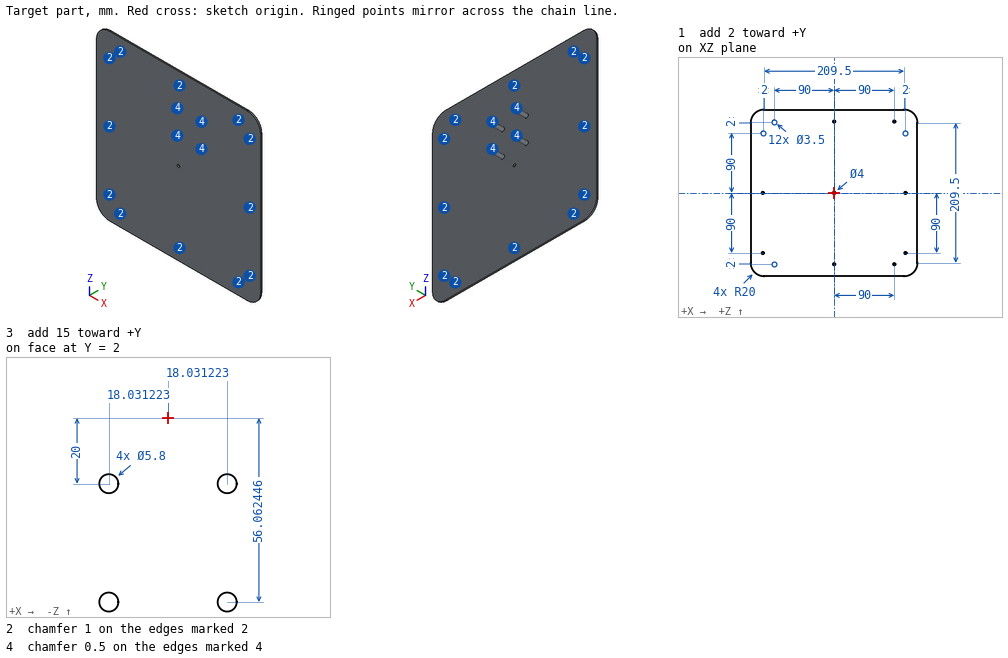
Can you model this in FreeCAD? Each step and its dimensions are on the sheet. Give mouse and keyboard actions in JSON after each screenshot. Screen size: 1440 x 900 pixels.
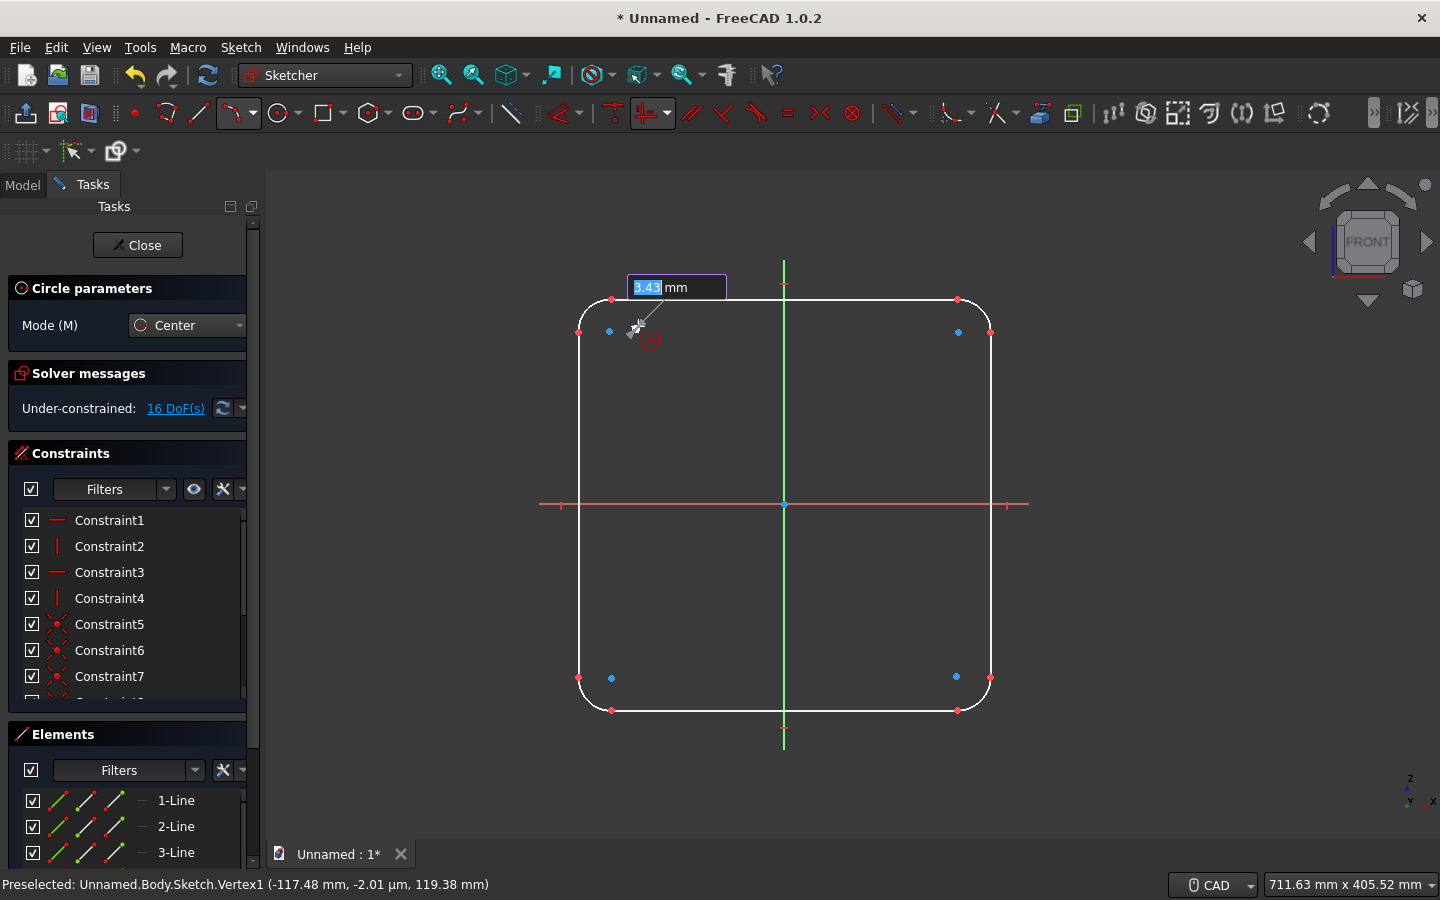
{"action": "type", "text": "3.5"}
{"action": "key", "text": "Return"}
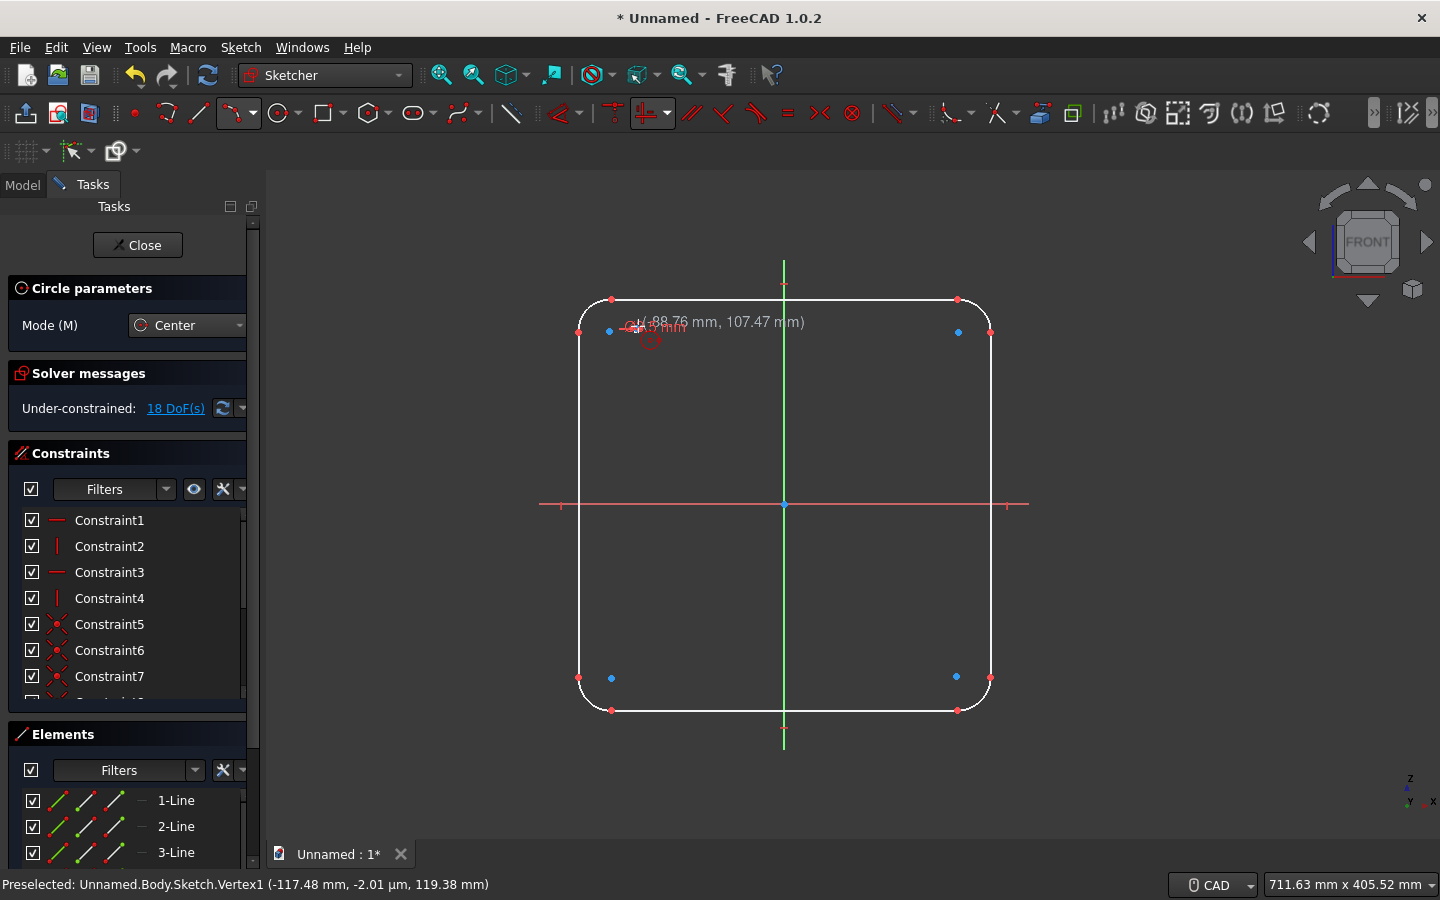
{"action": "scroll", "coordinate": [608, 356], "scroll_direction": "up", "scroll_amount": 11}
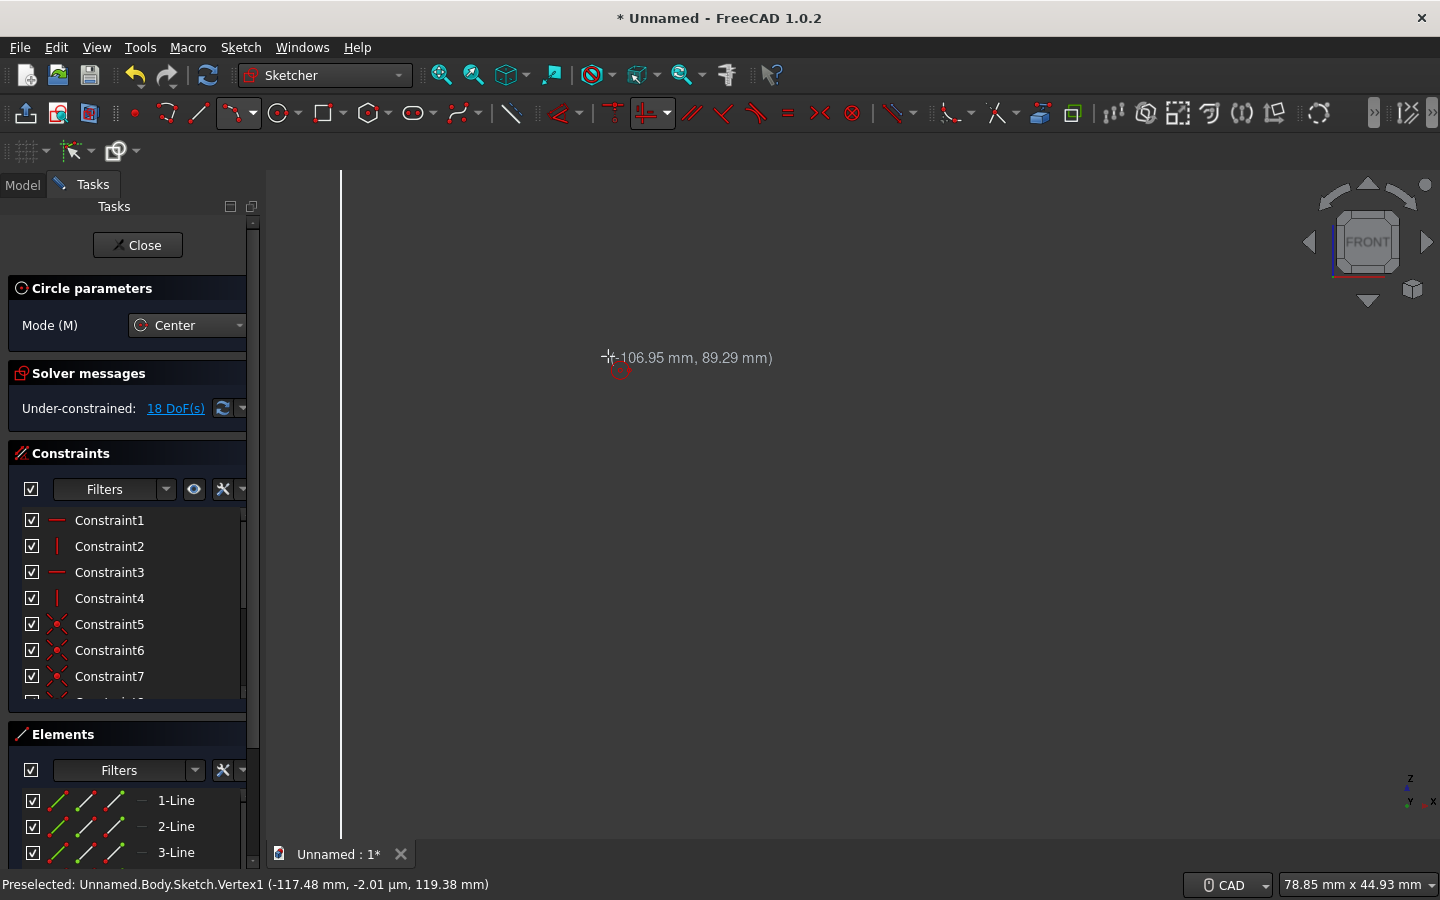
{"action": "scroll", "coordinate": [608, 357], "scroll_direction": "down", "scroll_amount": 11}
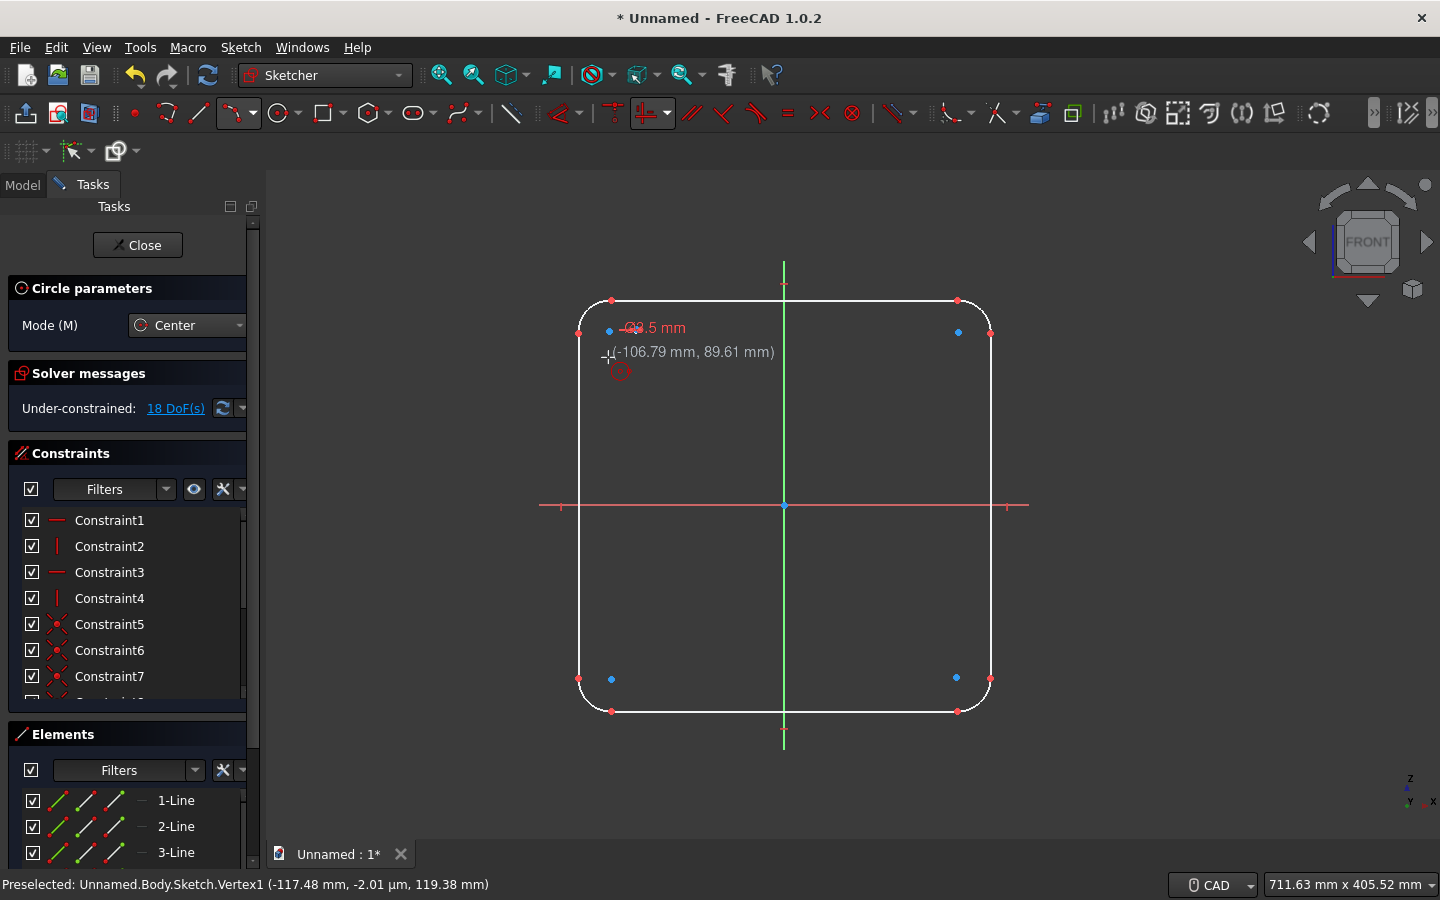
{"action": "left_click", "coordinate": [608, 357]}
{"action": "mouse_move", "coordinate": [610, 355]}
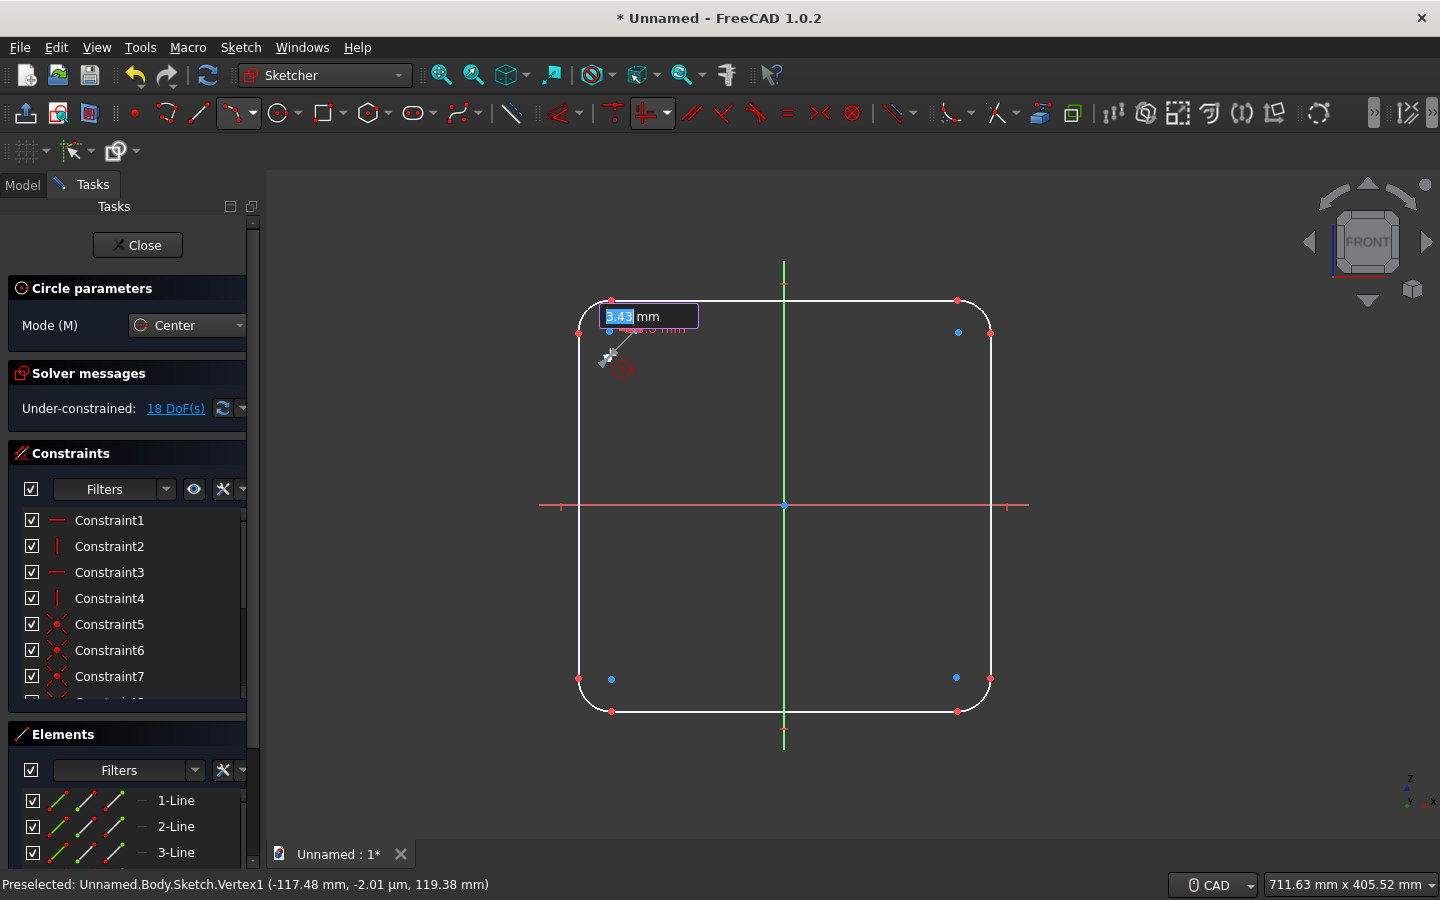
{"action": "type", "text": "3.5"}
{"action": "key", "text": "Return"}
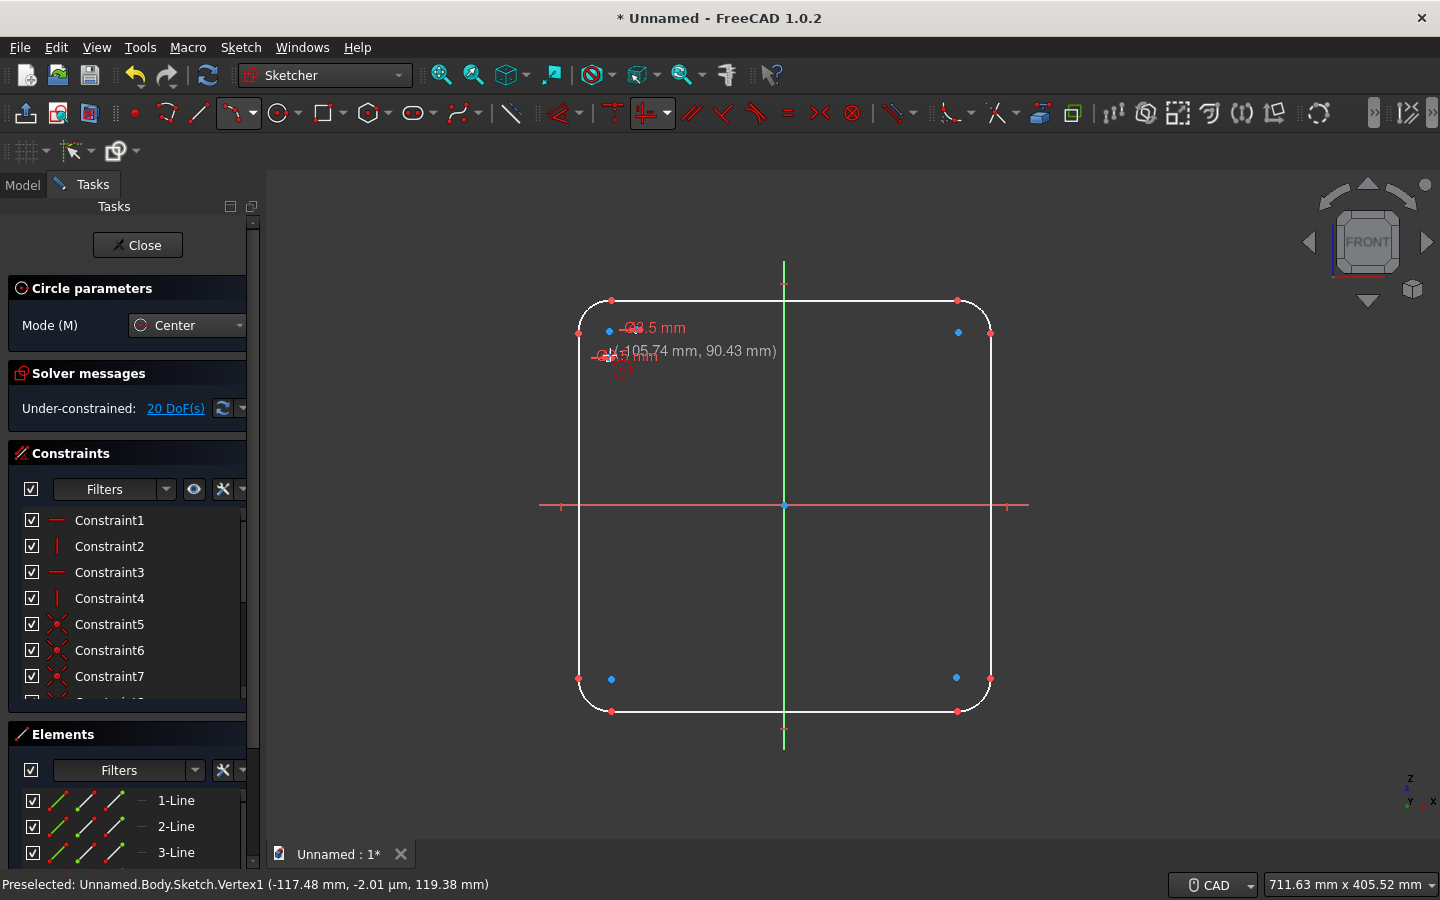
{"action": "scroll", "coordinate": [784, 329], "scroll_direction": "up", "scroll_amount": 11}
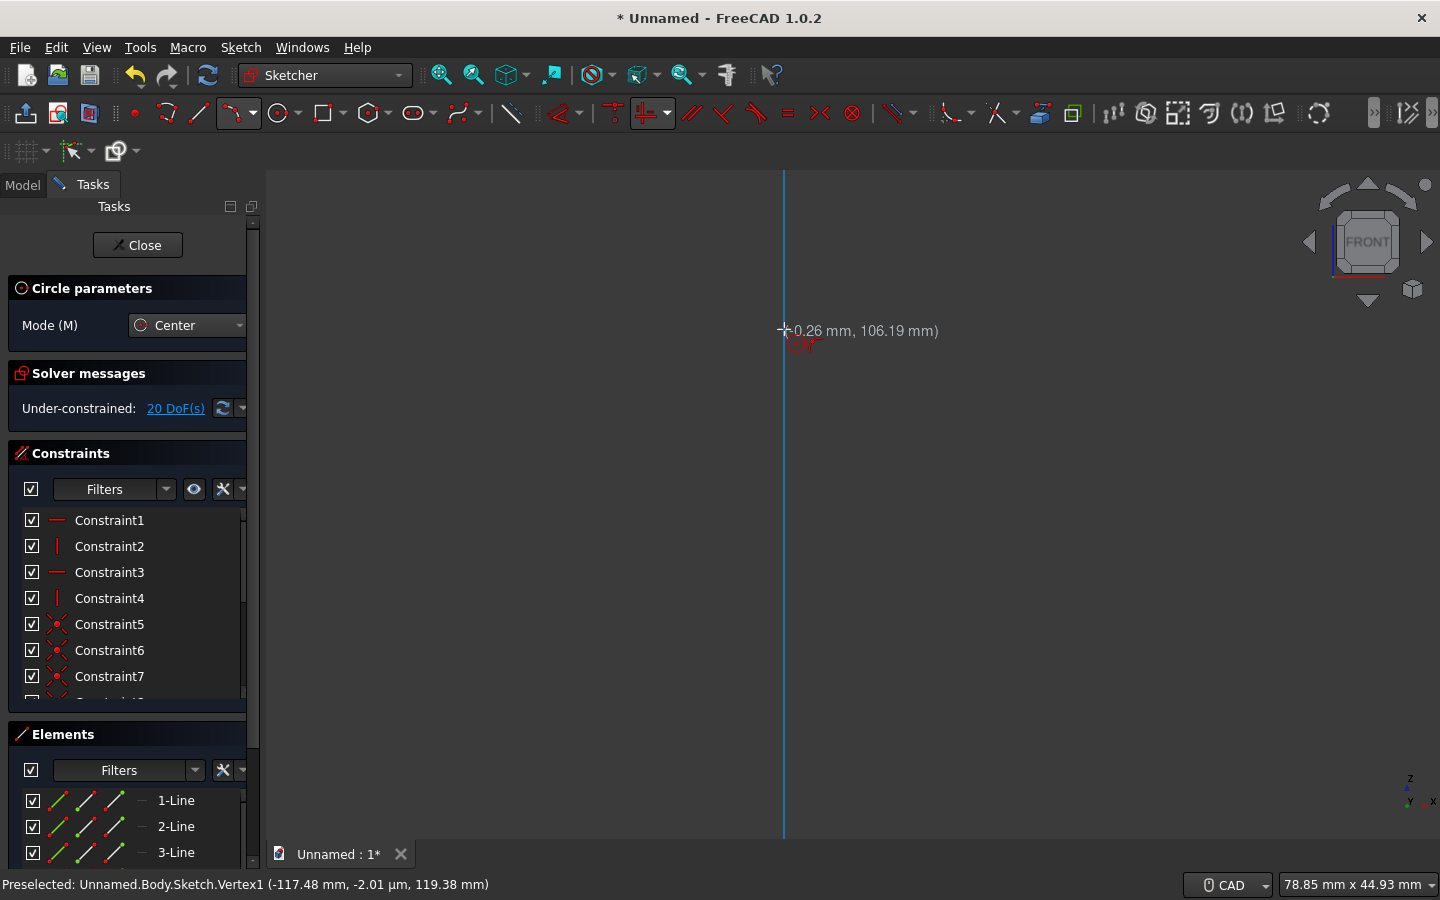
{"action": "scroll", "coordinate": [785, 328], "scroll_direction": "down", "scroll_amount": 11}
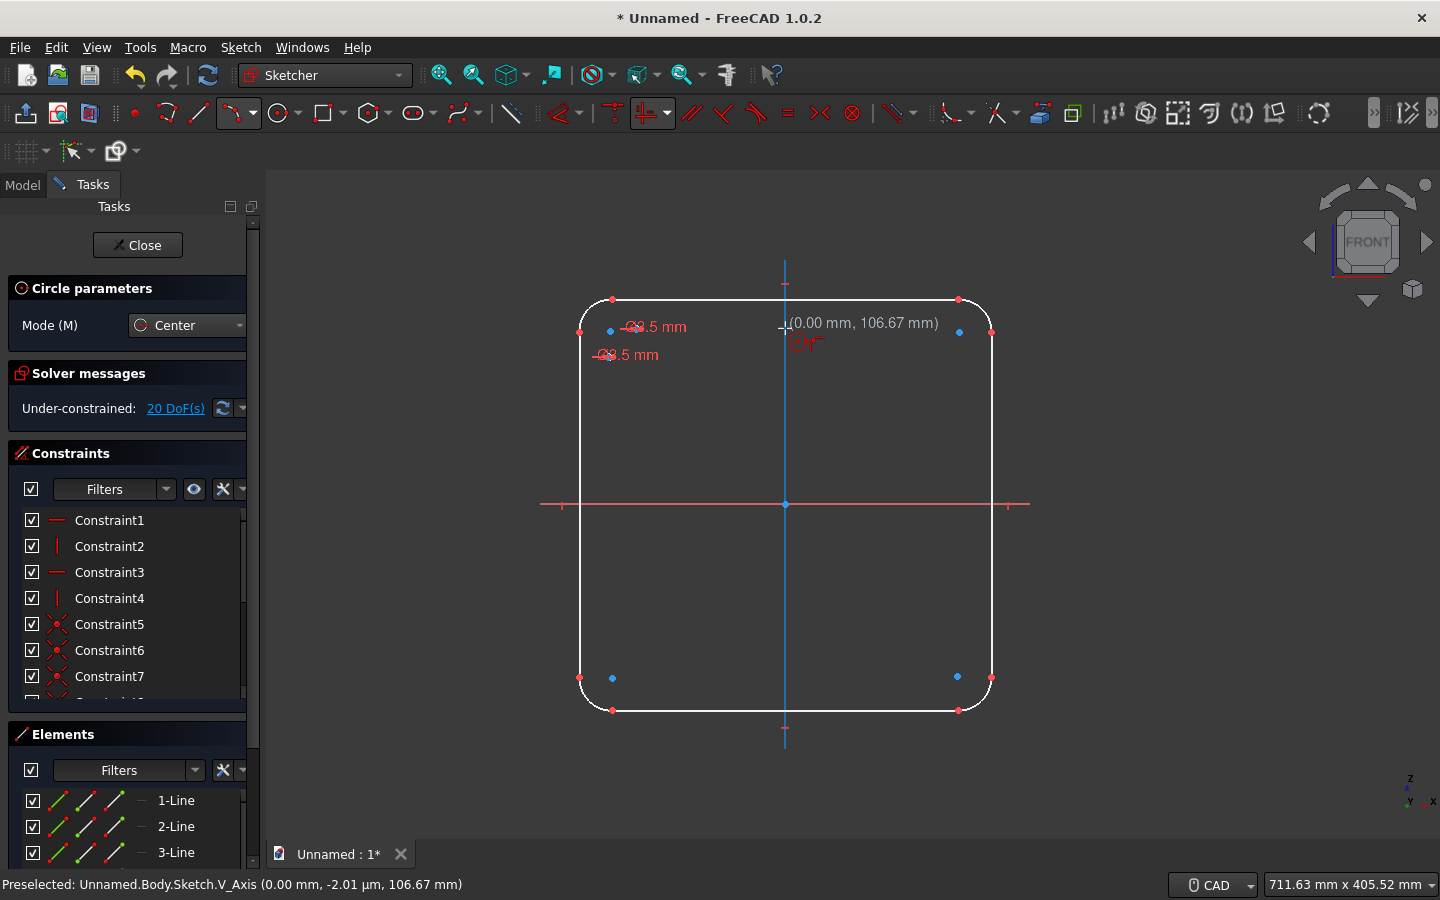
{"action": "left_click", "coordinate": [785, 328]}